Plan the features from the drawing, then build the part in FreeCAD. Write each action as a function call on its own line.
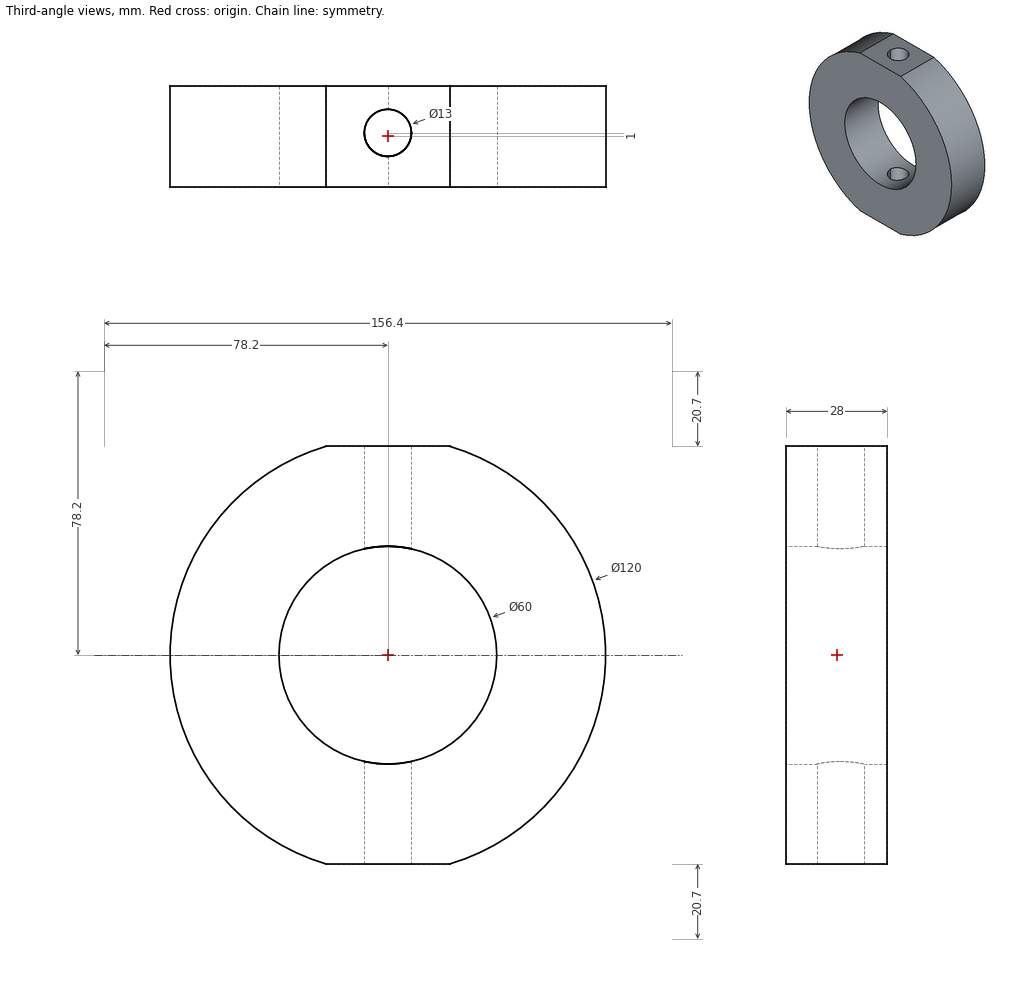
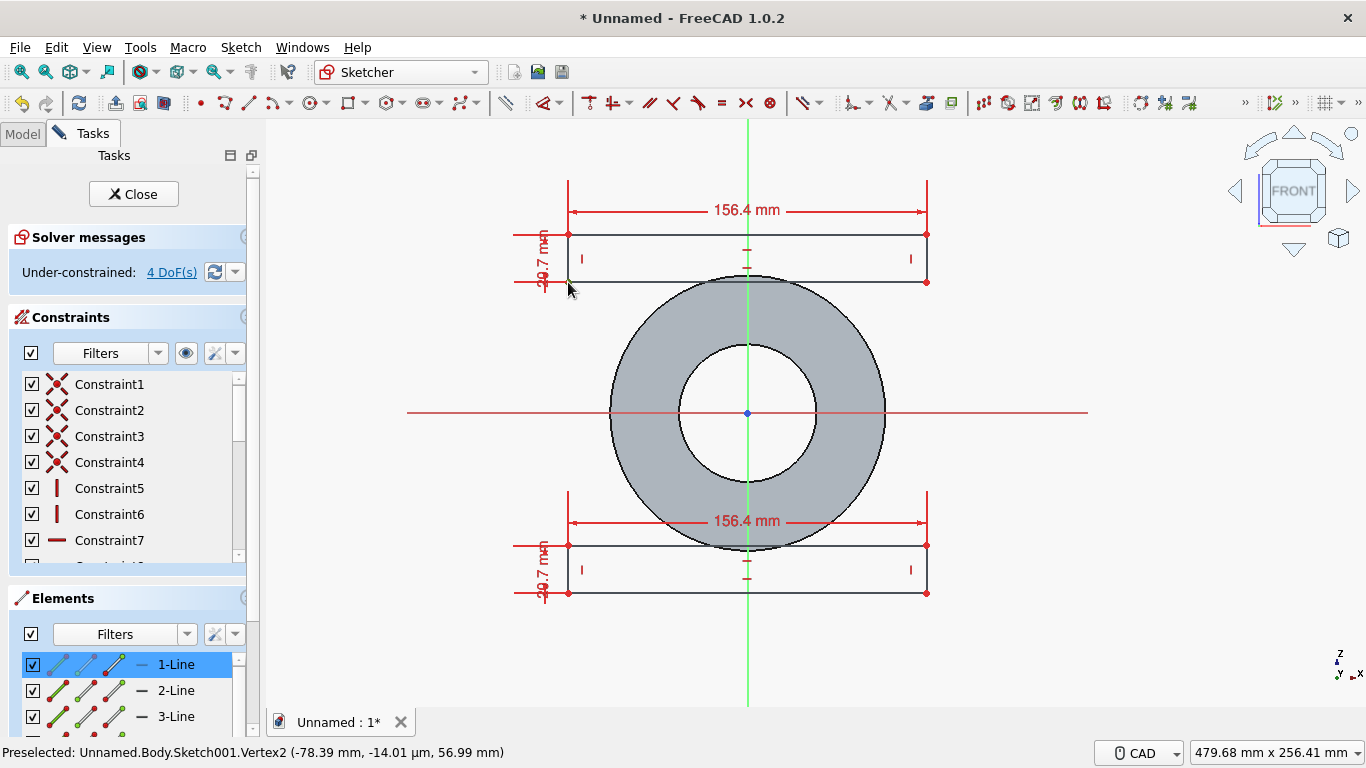
click(568, 546)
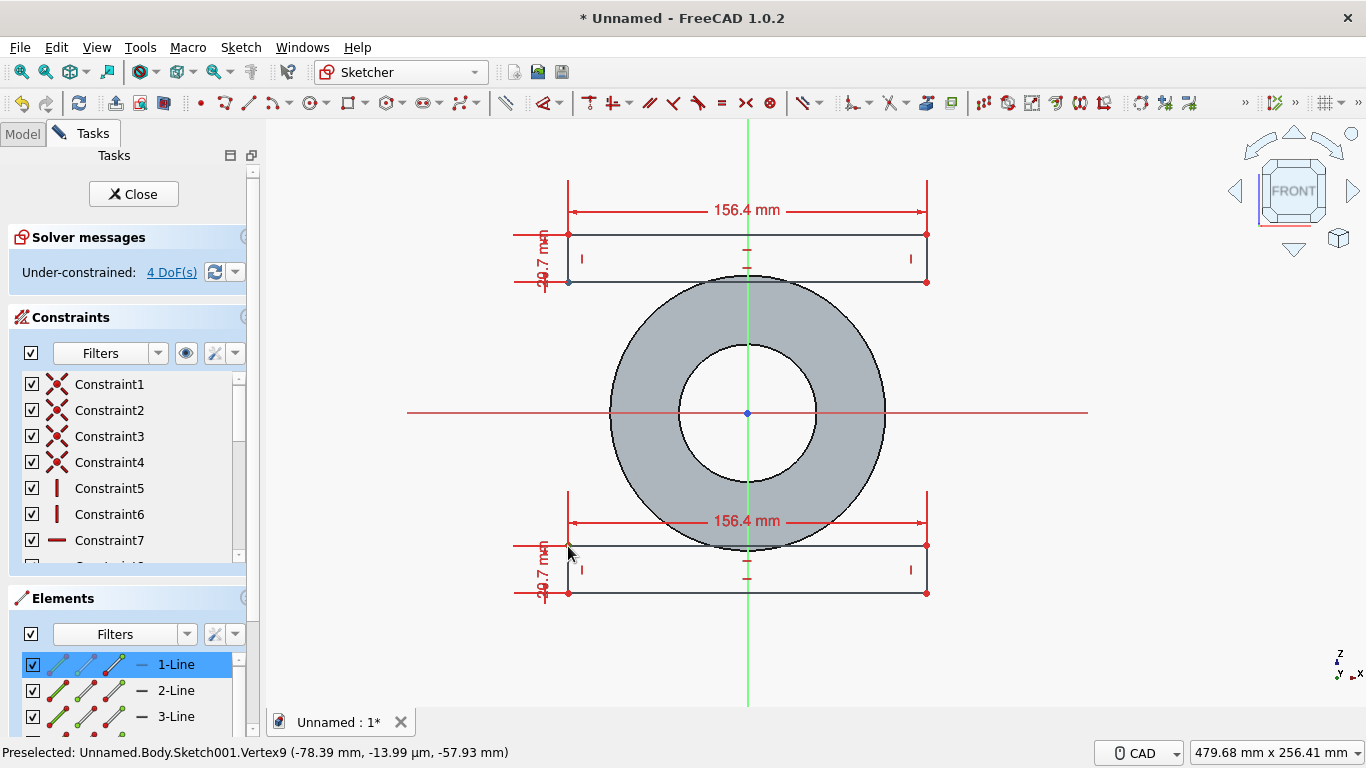
click(424, 413)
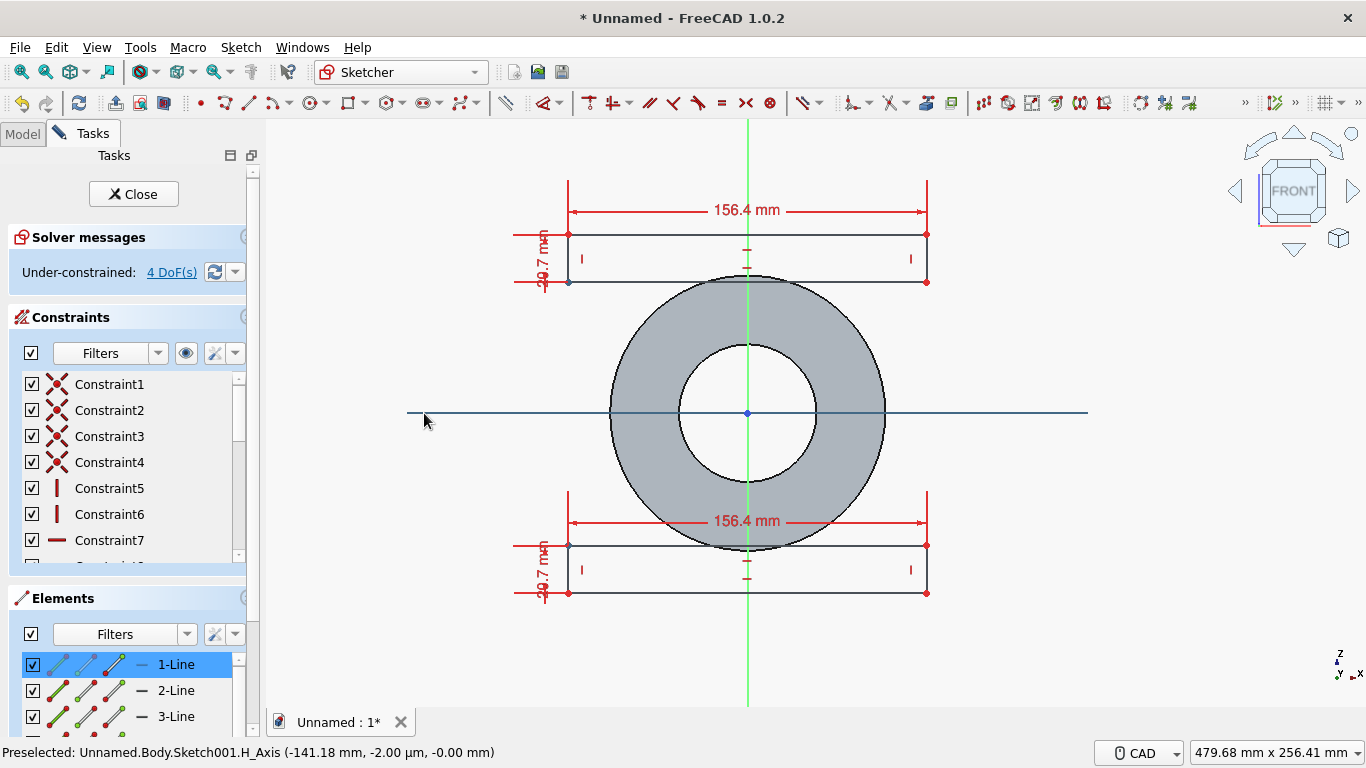
click(746, 104)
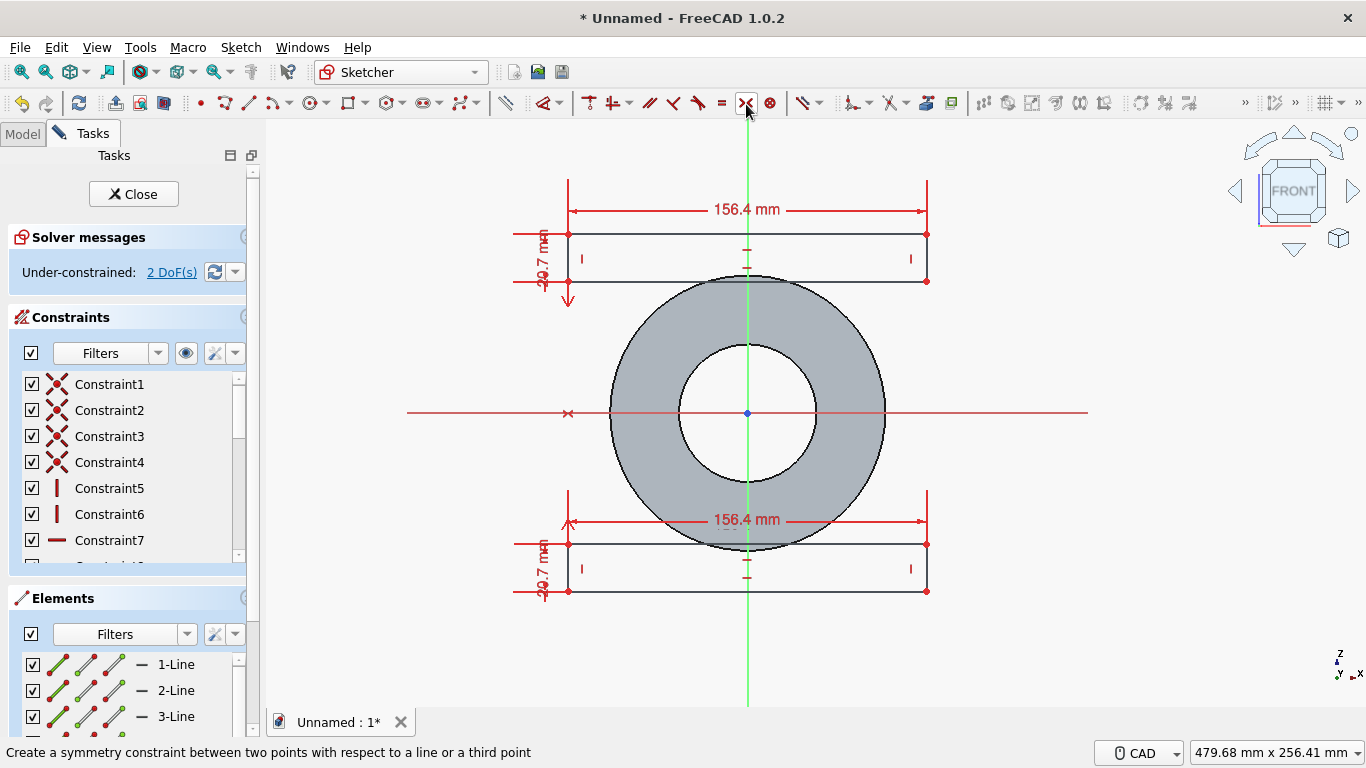
click(544, 104)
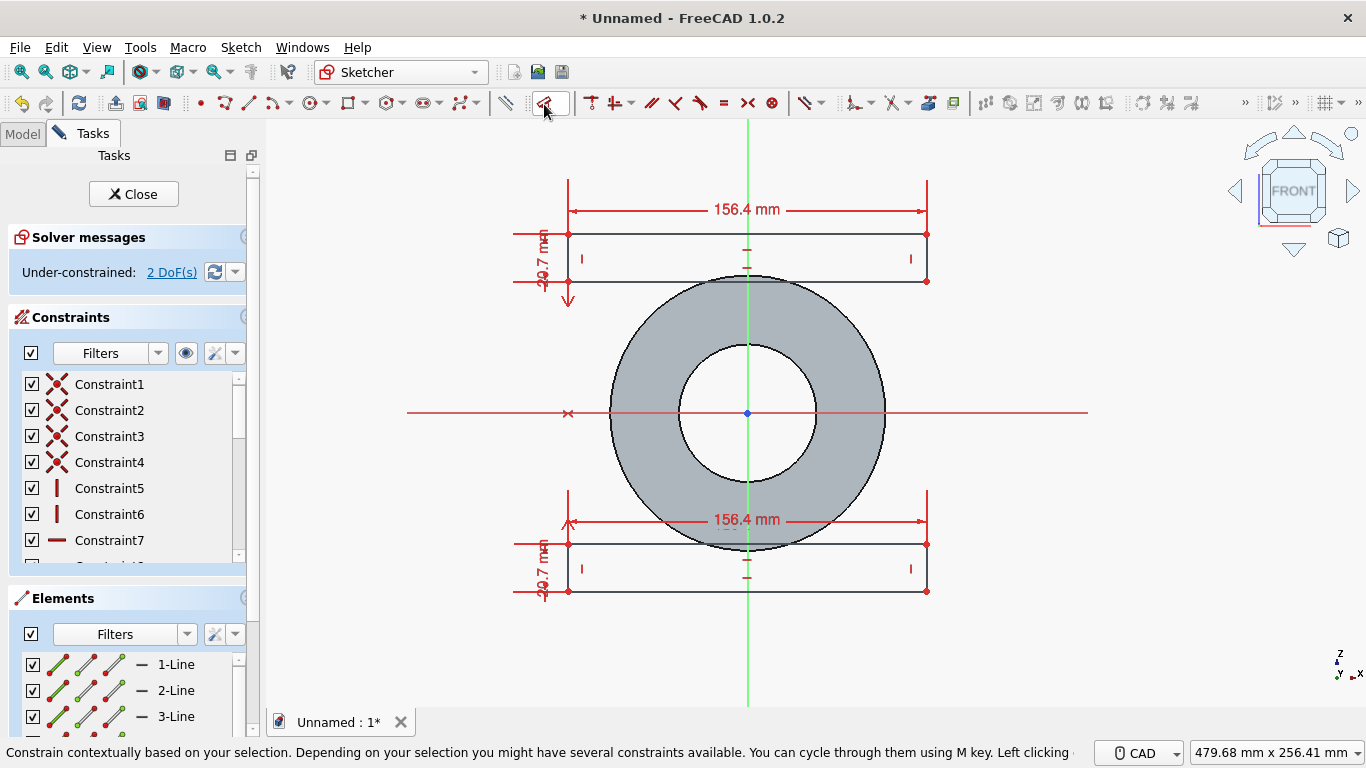
click(568, 234)
click(658, 200)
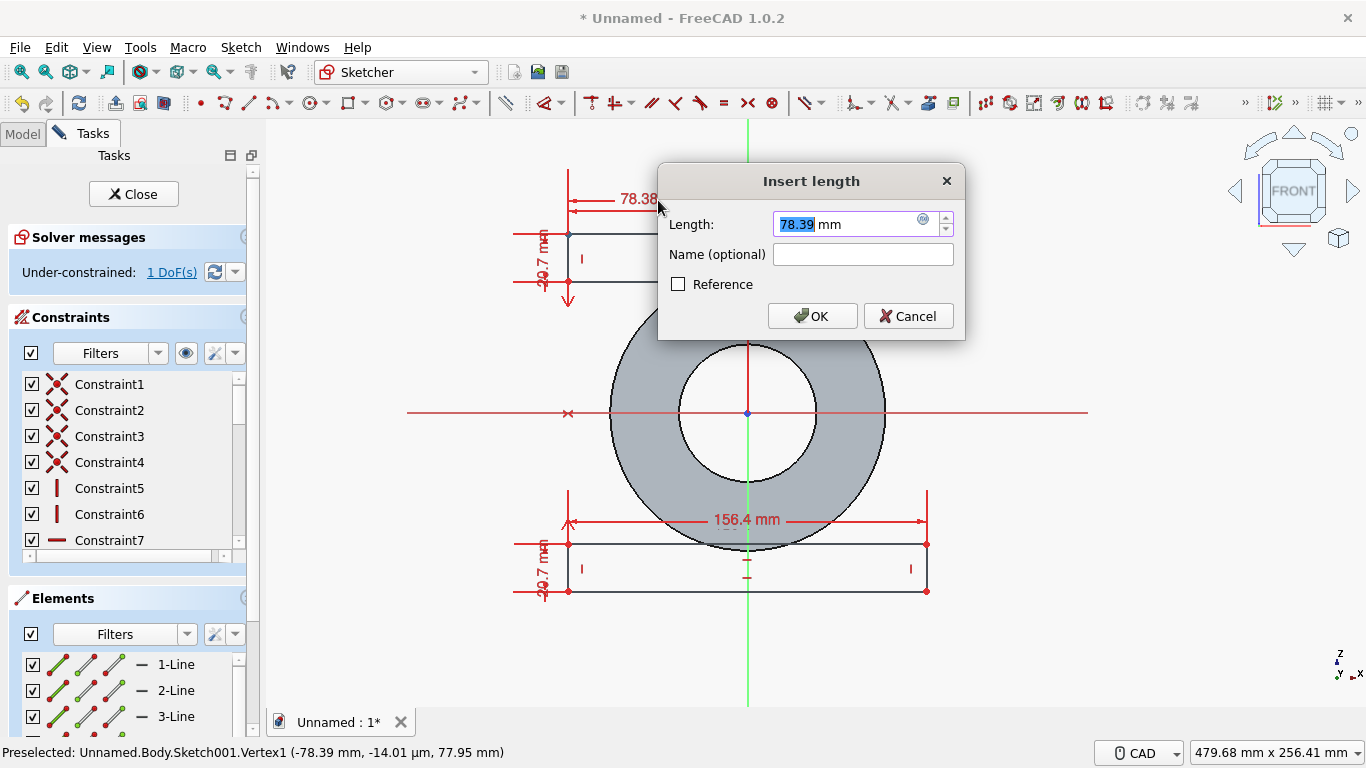
text(78.2)
key(Return)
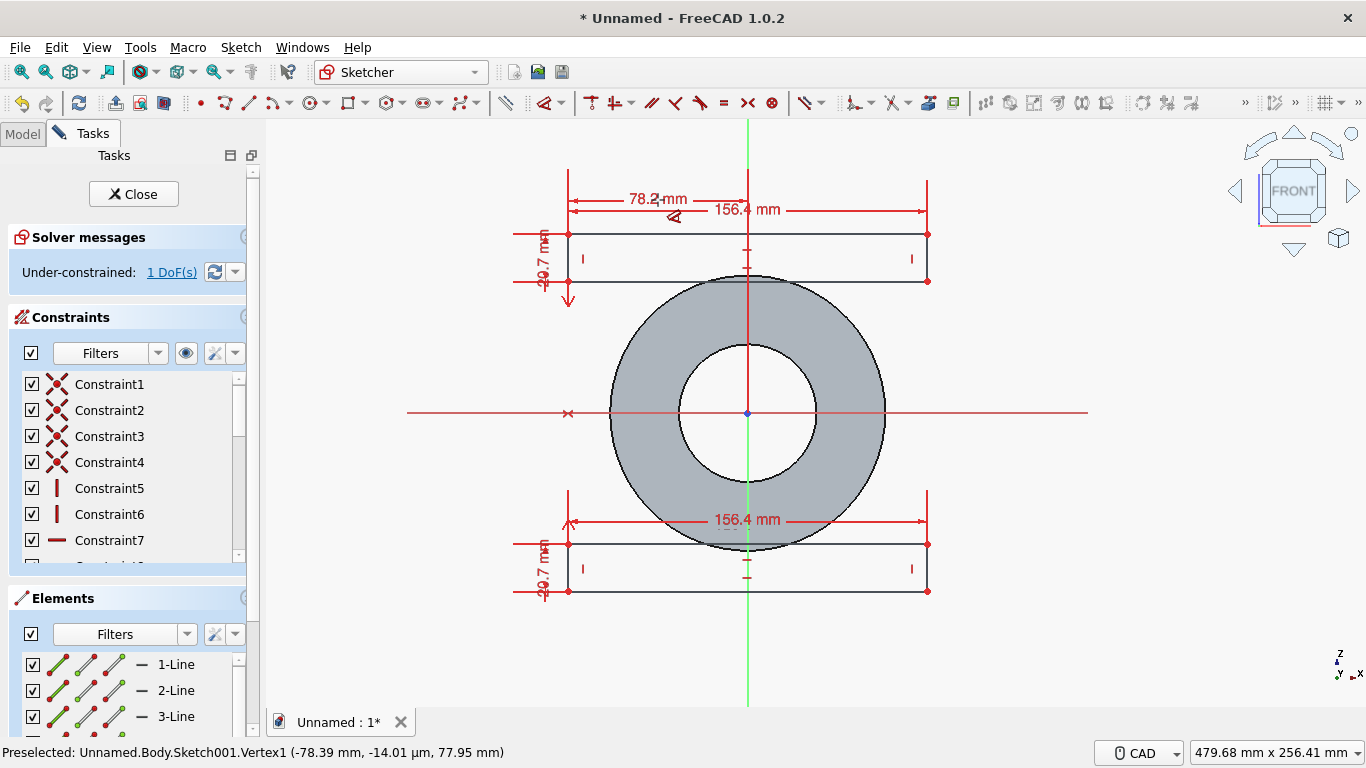
click(568, 234)
click(534, 324)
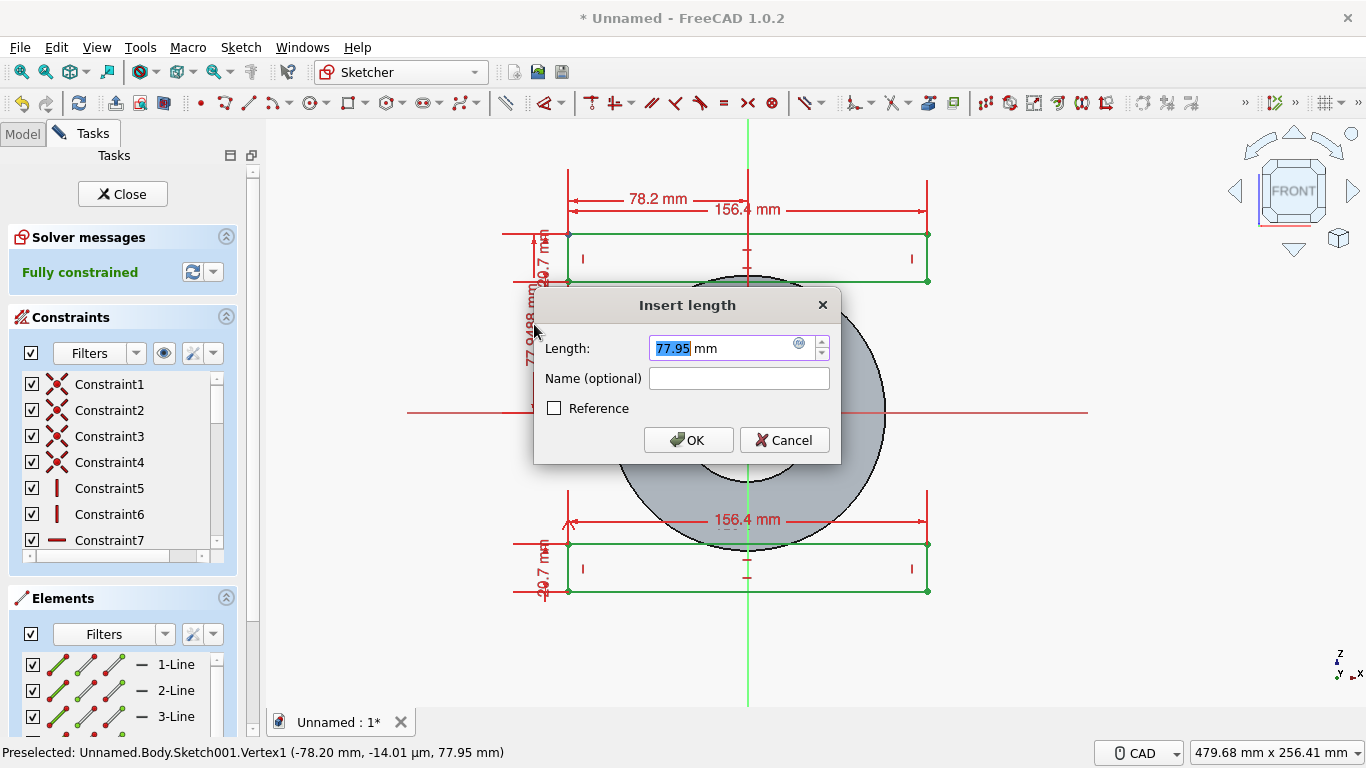
text(78.2)
key(Return)
key(Escape)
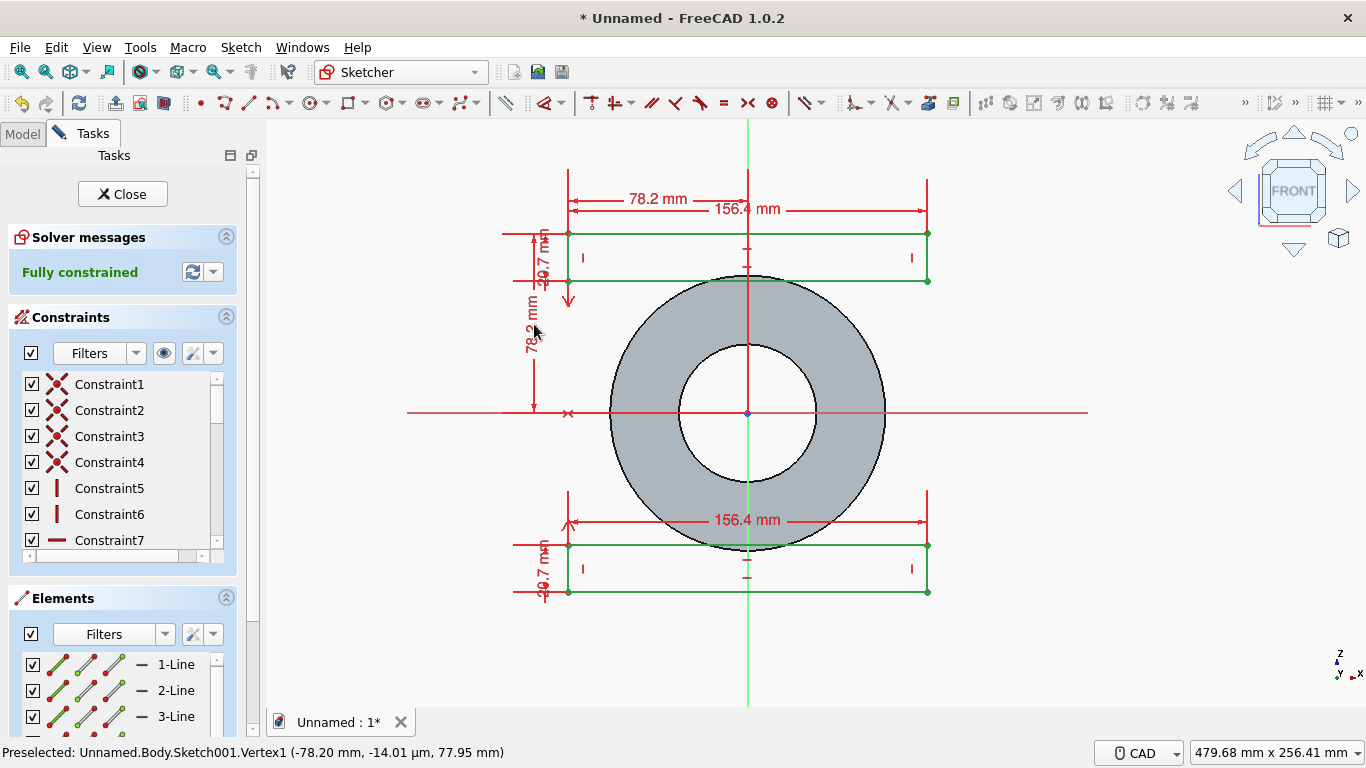
click(123, 194)